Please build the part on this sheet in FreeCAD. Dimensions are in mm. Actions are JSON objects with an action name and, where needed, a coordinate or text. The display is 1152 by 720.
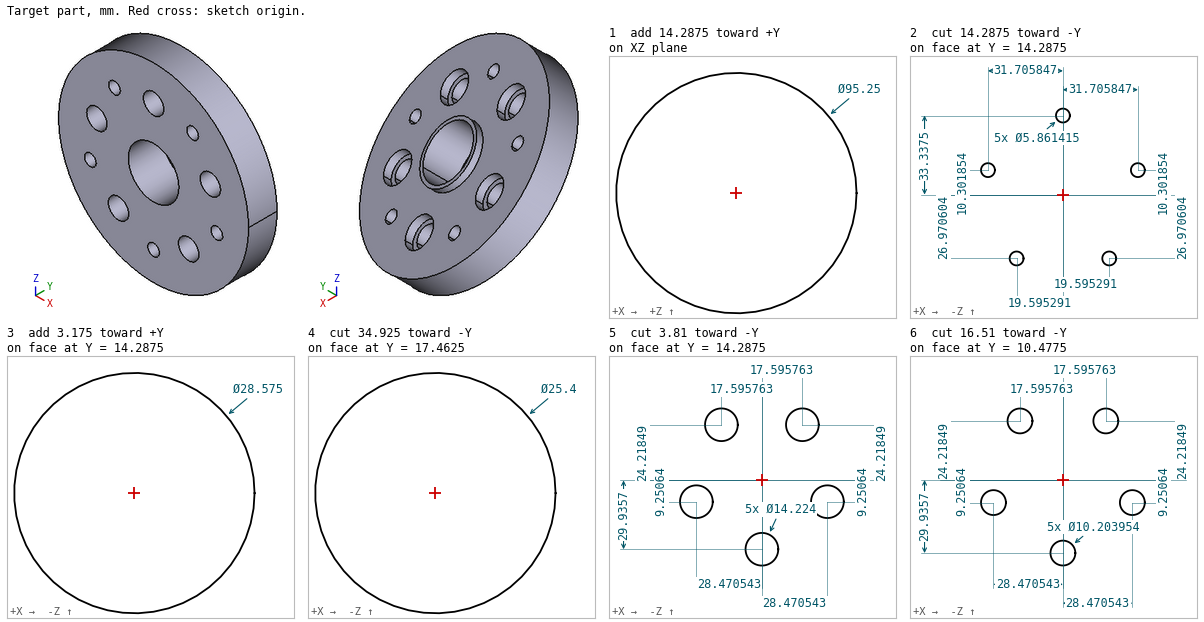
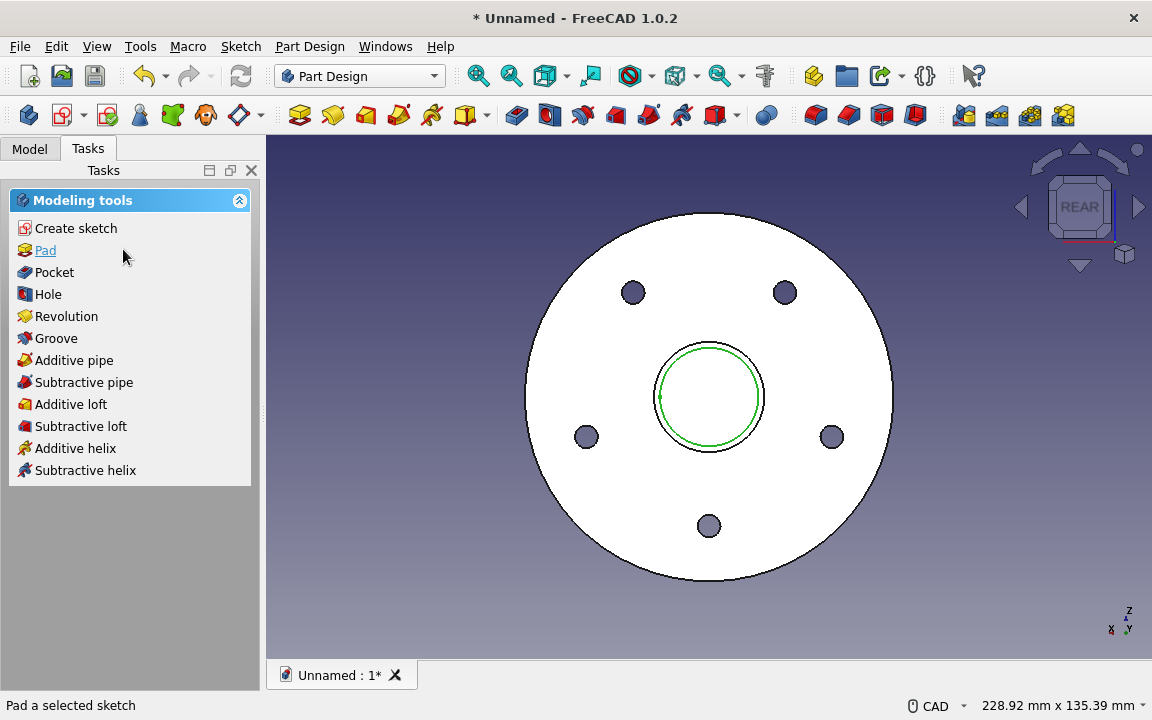
{"action": "left_click", "coordinate": [517, 116]}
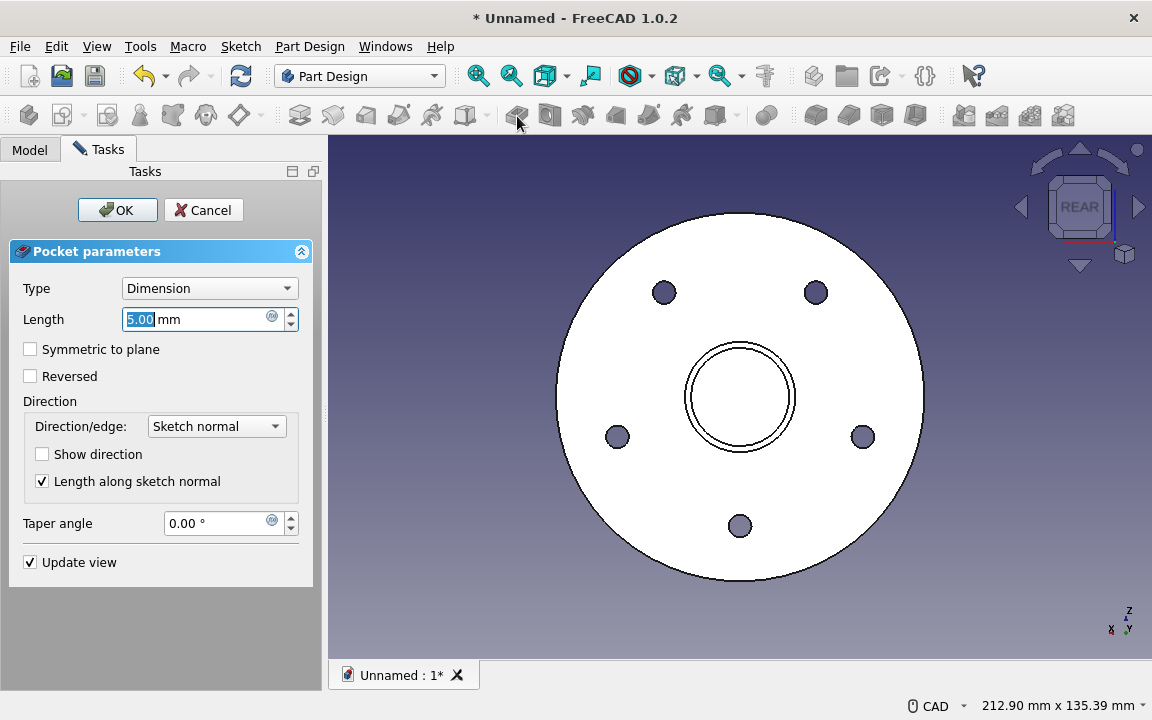
{"action": "type", "text": "34.925"}
{"action": "key", "text": "Tab"}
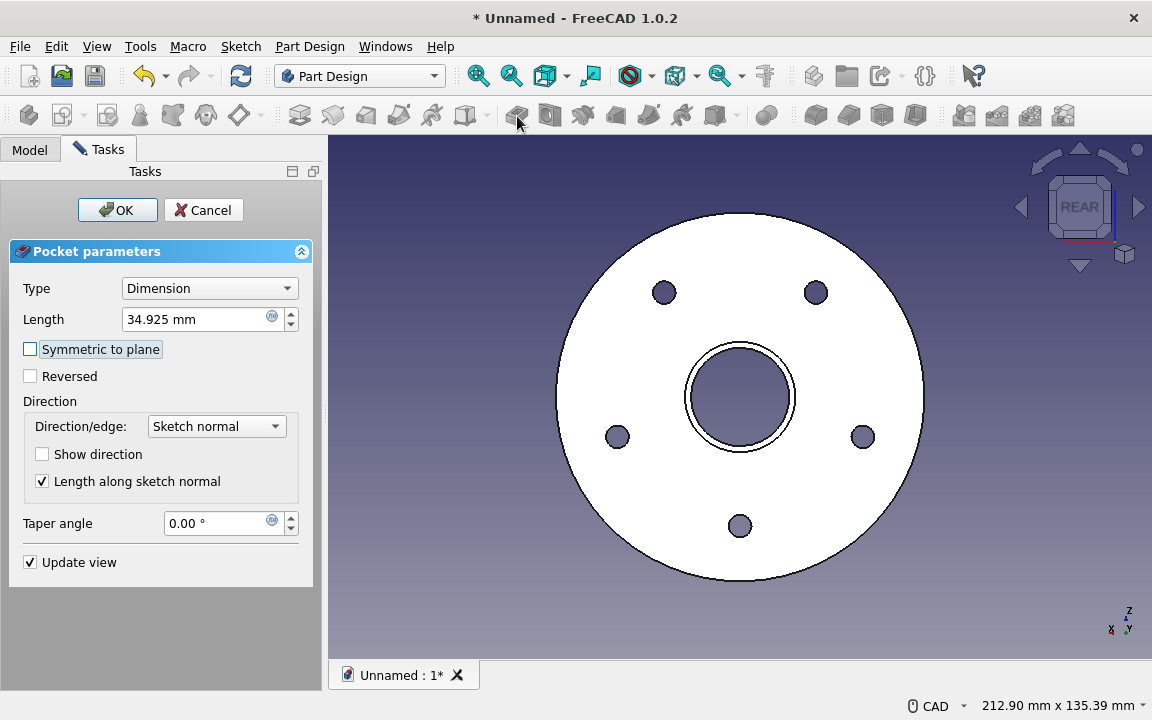
{"action": "left_click", "coordinate": [118, 210]}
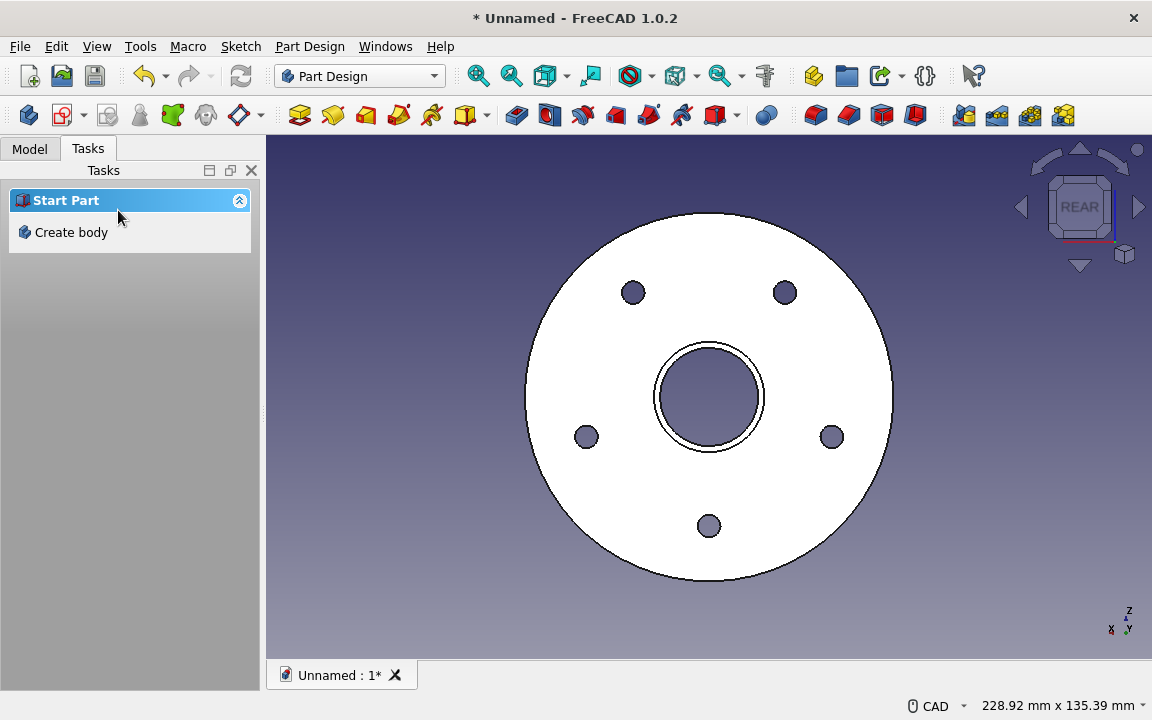
{"action": "left_click", "coordinate": [709, 291]}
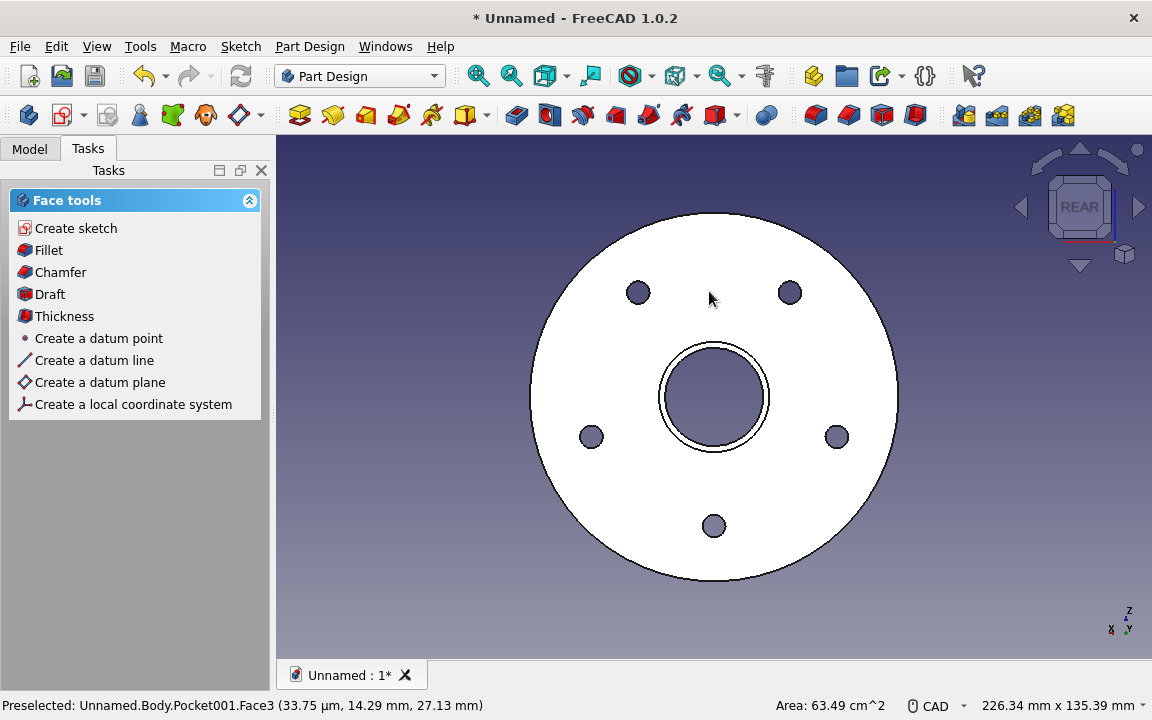
{"action": "left_click", "coordinate": [62, 116]}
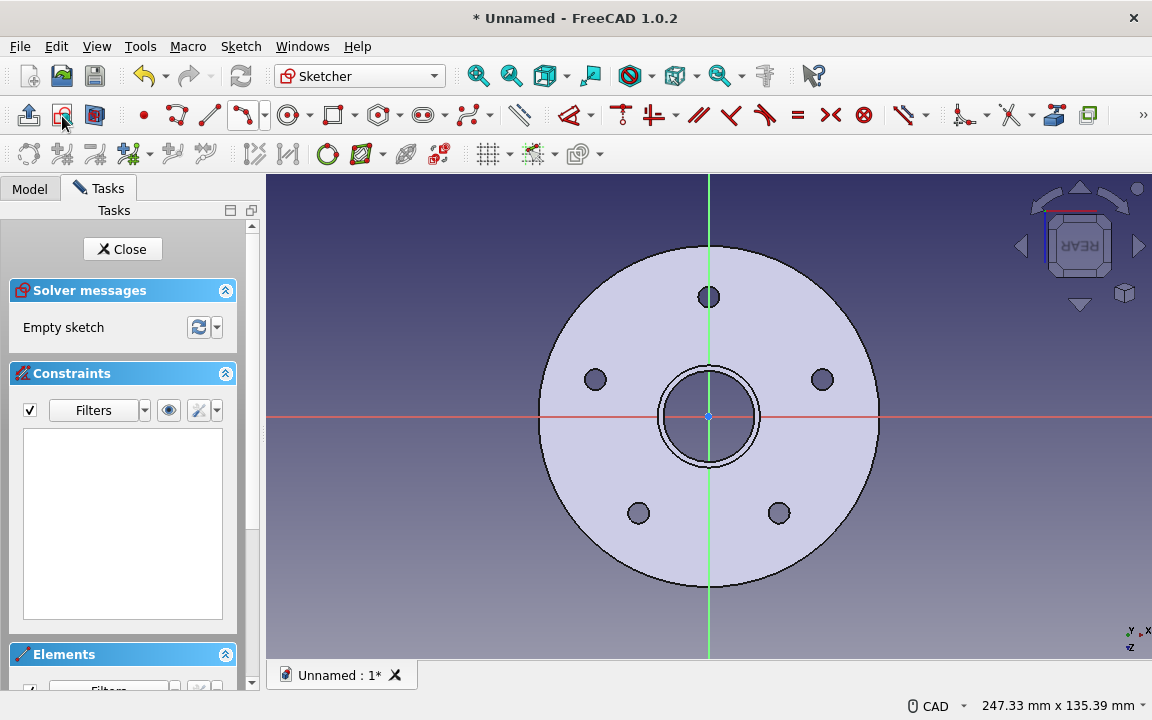
{"action": "left_click", "coordinate": [288, 116]}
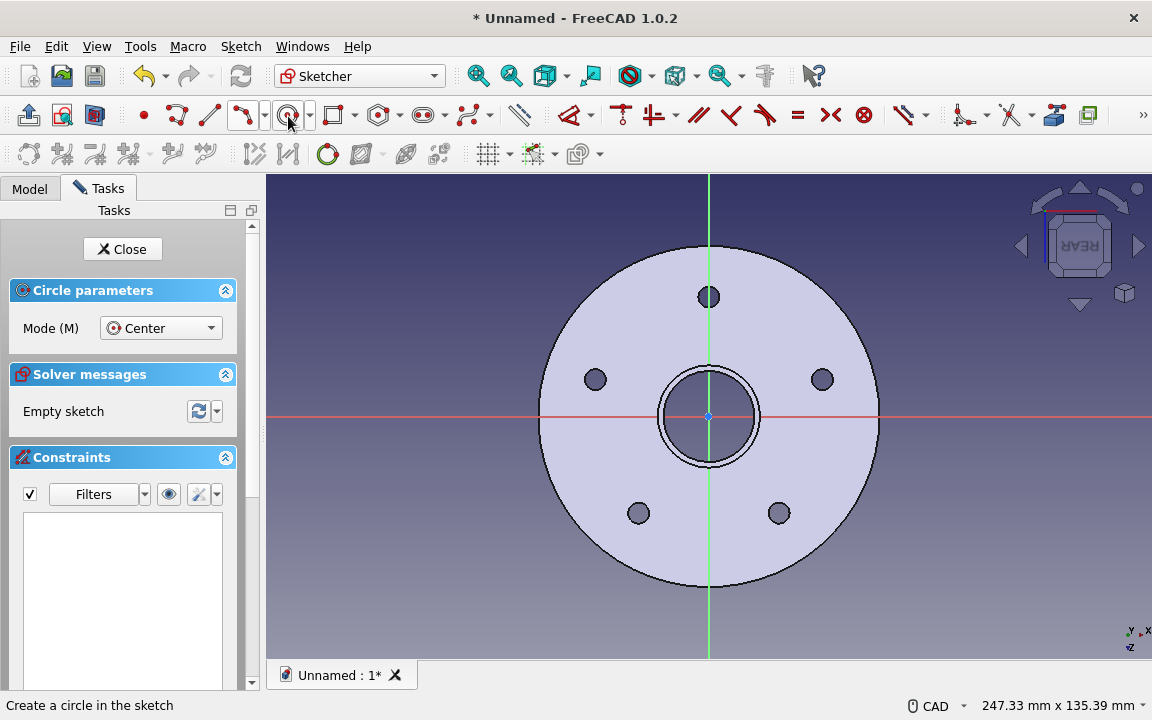
{"action": "left_click", "coordinate": [709, 524]}
{"action": "mouse_move", "coordinate": [727, 506]}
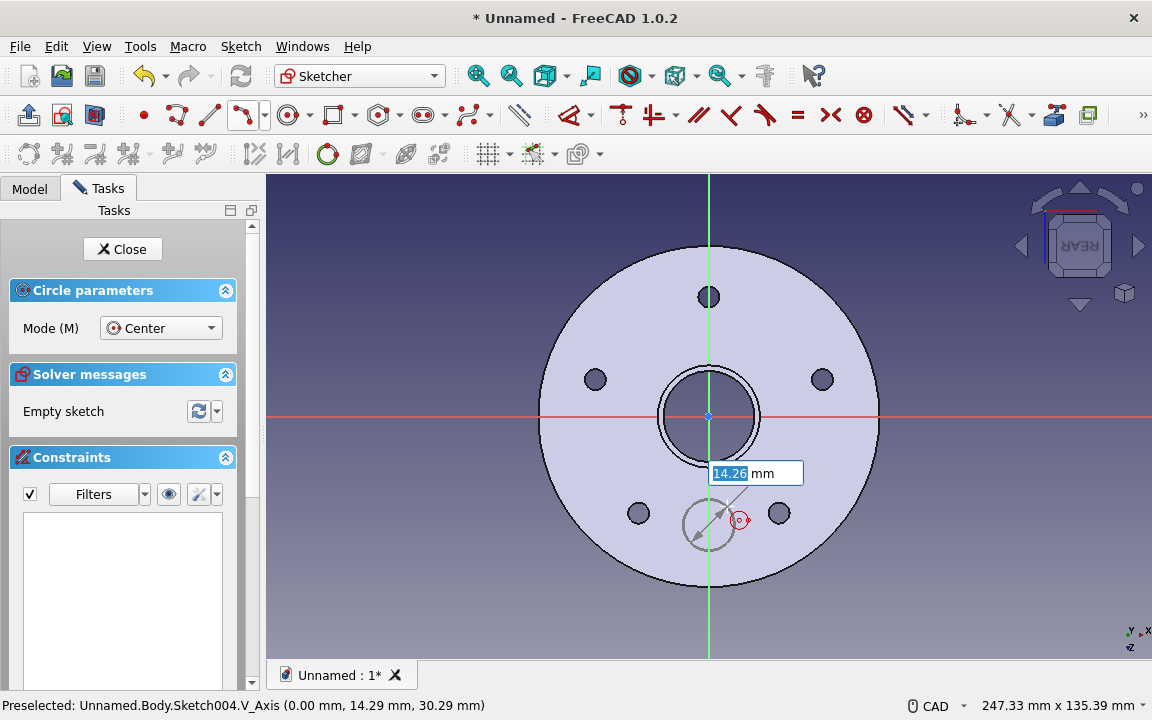
{"action": "type", "text": "14.224"}
{"action": "key", "text": "Return"}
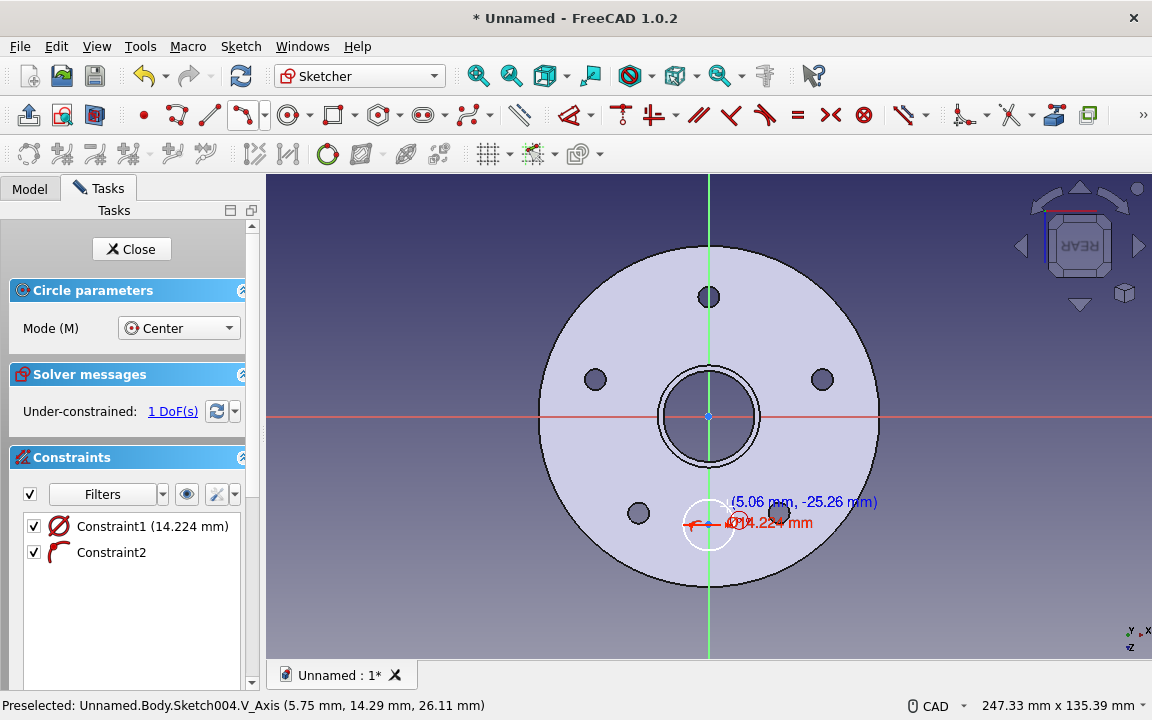
{"action": "left_click", "coordinate": [607, 450]}
{"action": "mouse_move", "coordinate": [625, 432]}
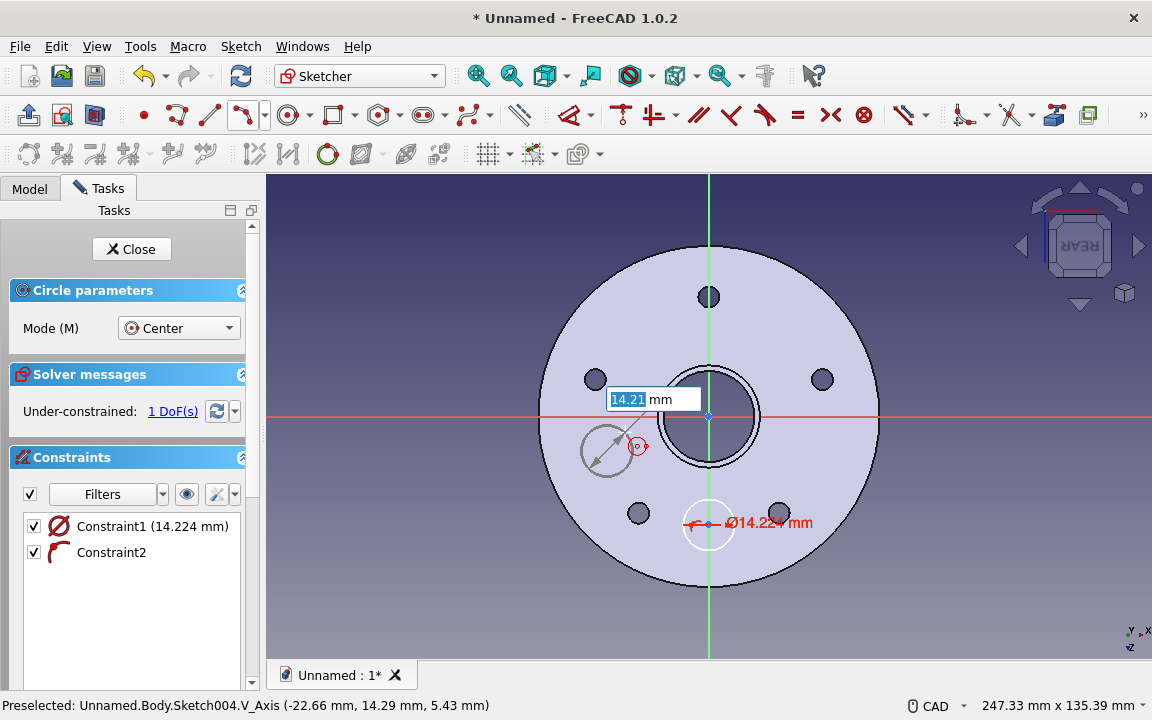
{"action": "type", "text": "14.224"}
{"action": "key", "text": "Return"}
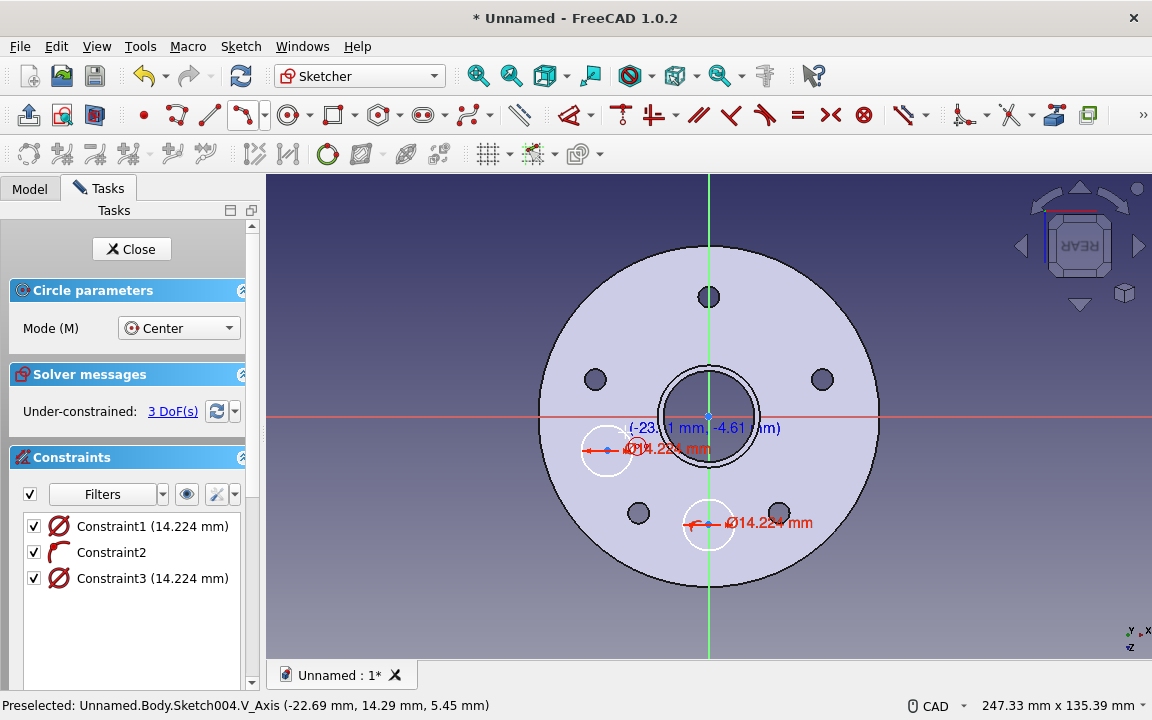
{"action": "left_click", "coordinate": [646, 330]}
{"action": "mouse_move", "coordinate": [664, 312]}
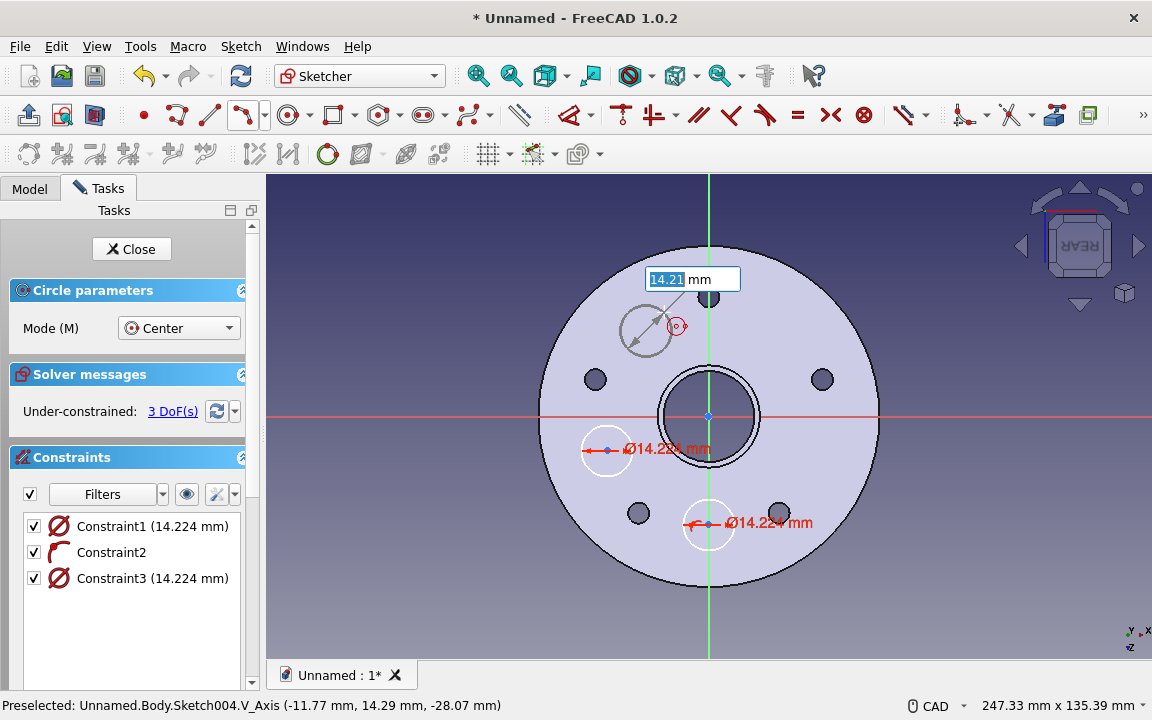
{"action": "type", "text": "14.224"}
{"action": "key", "text": "Return"}